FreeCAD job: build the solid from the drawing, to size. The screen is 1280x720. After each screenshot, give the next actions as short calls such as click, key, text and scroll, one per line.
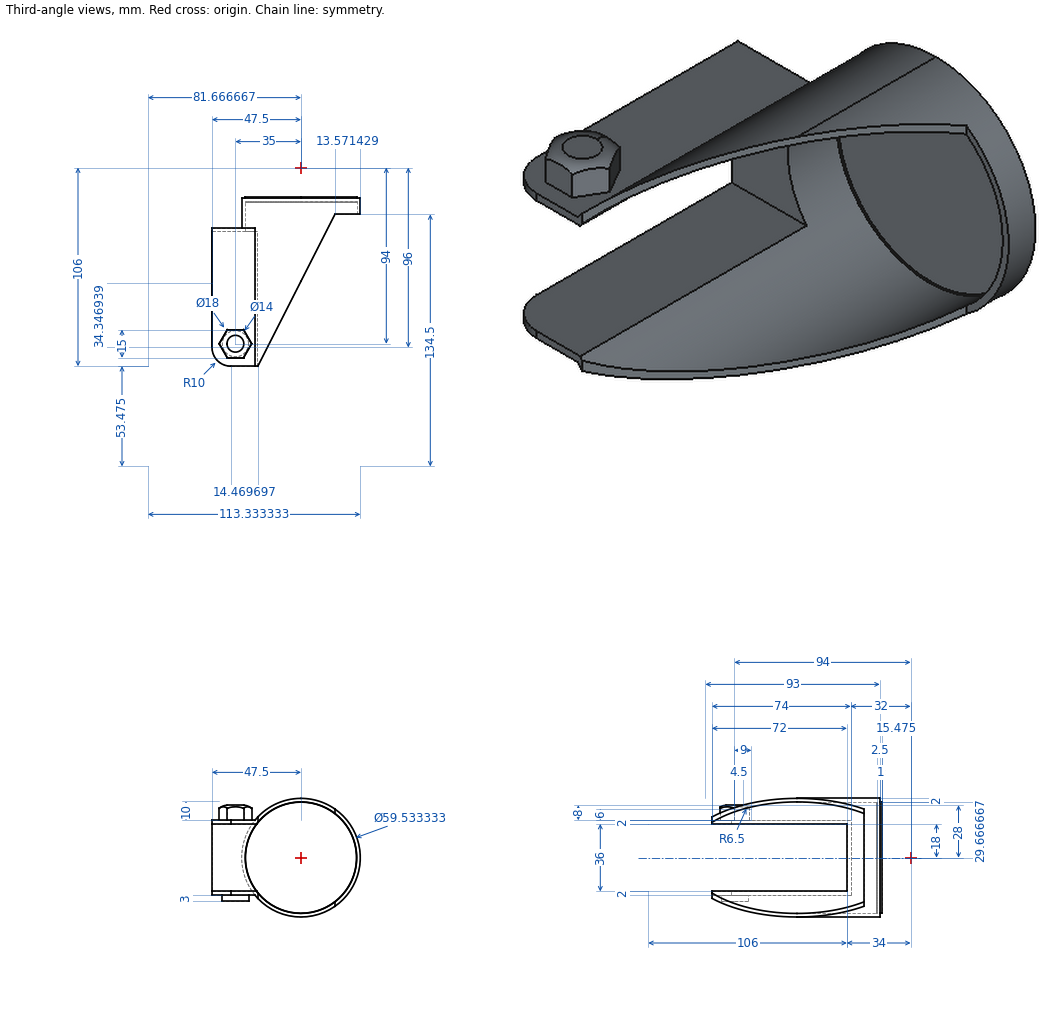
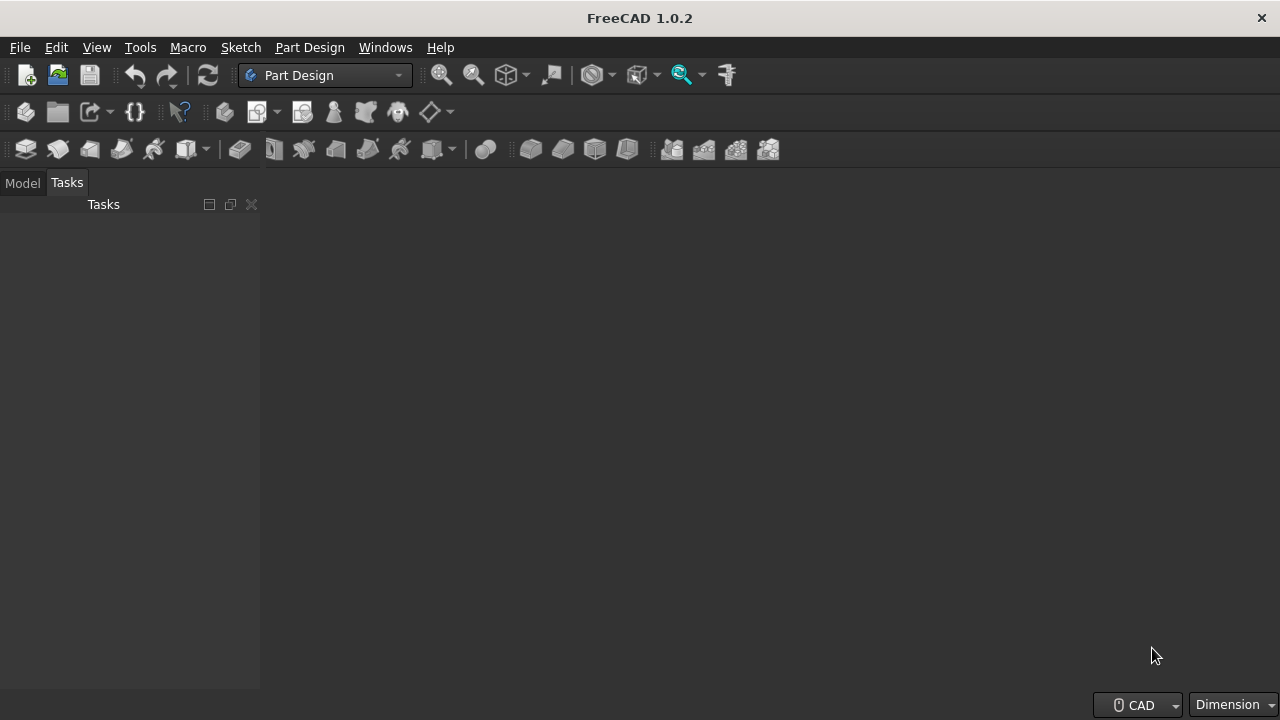
key(ctrl+n)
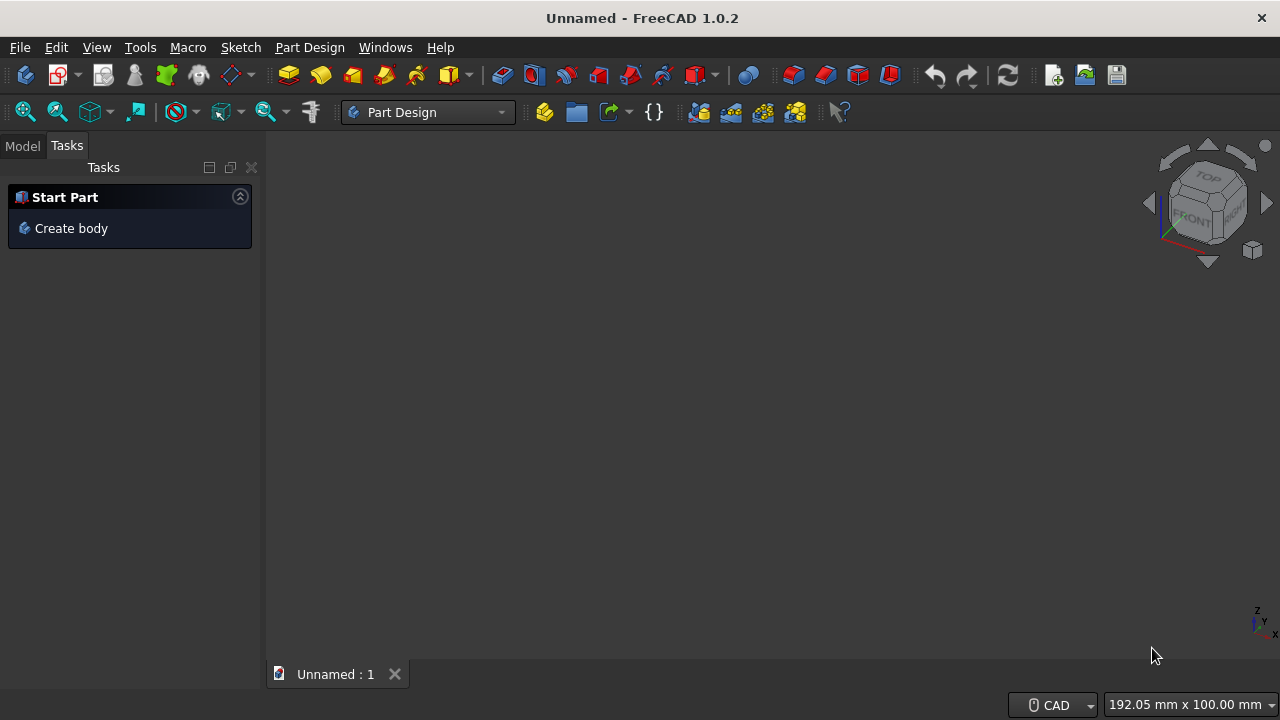
click(58, 76)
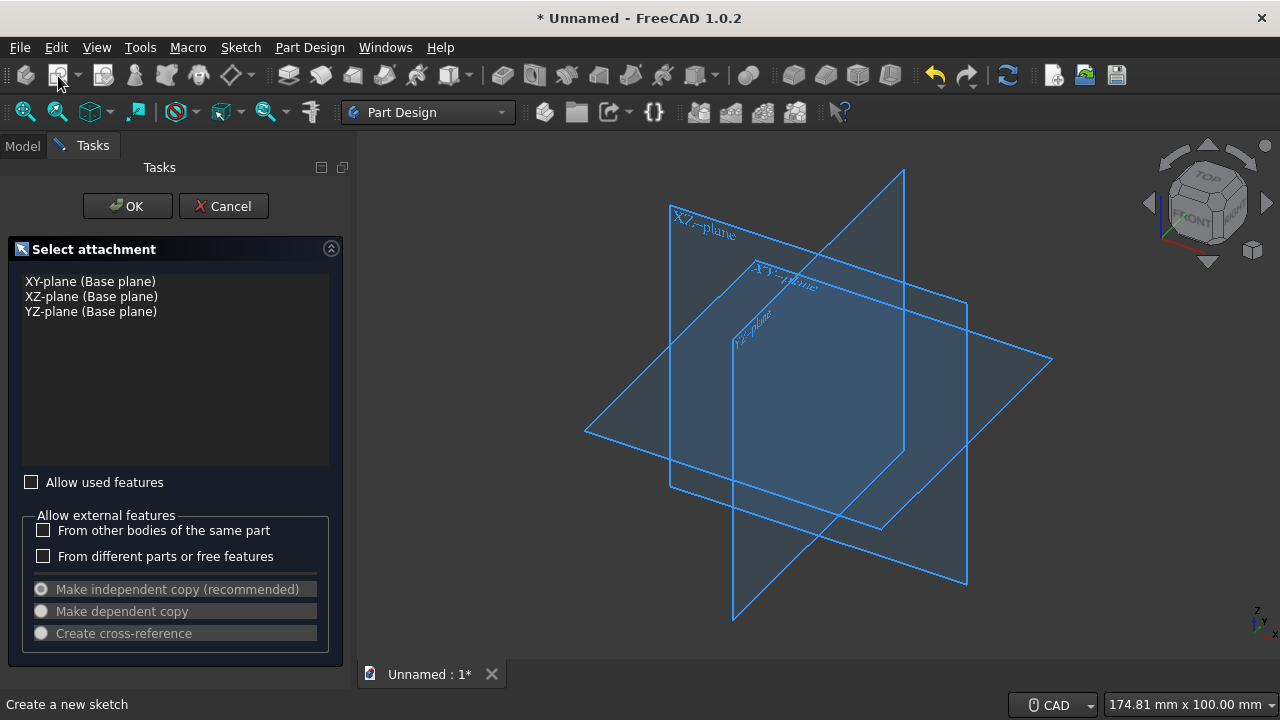
click(82, 312)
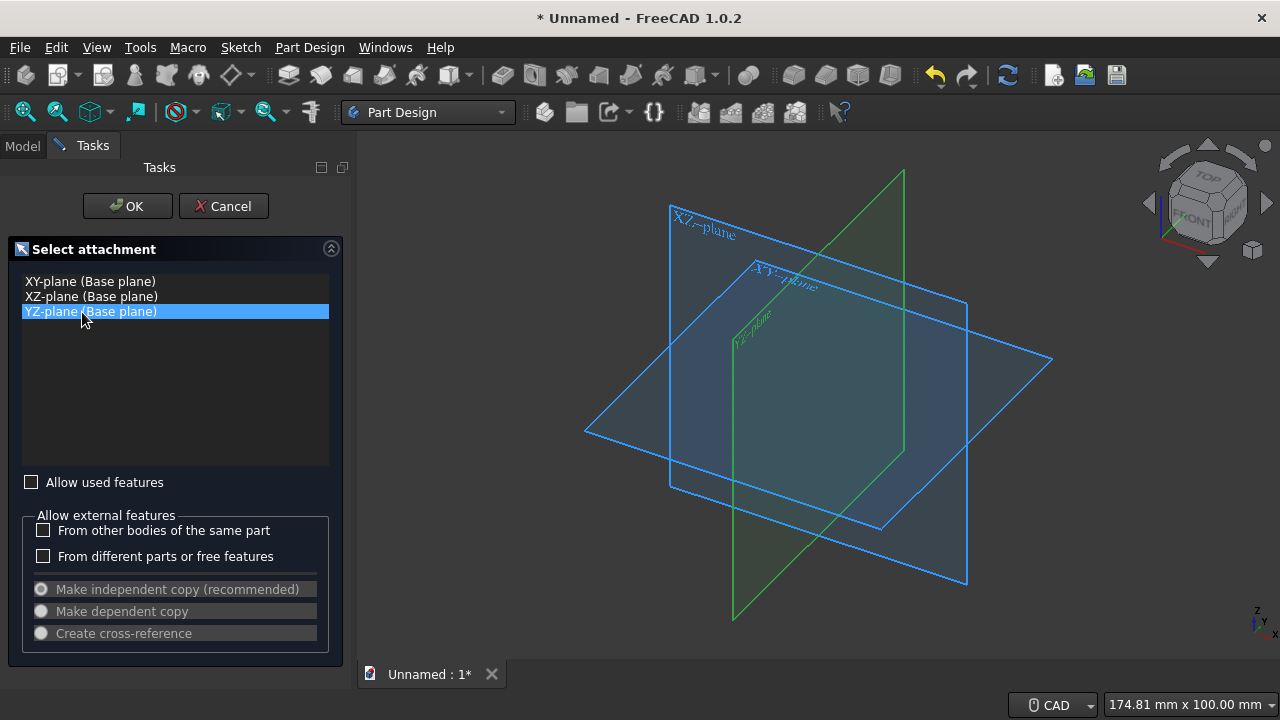
click(128, 206)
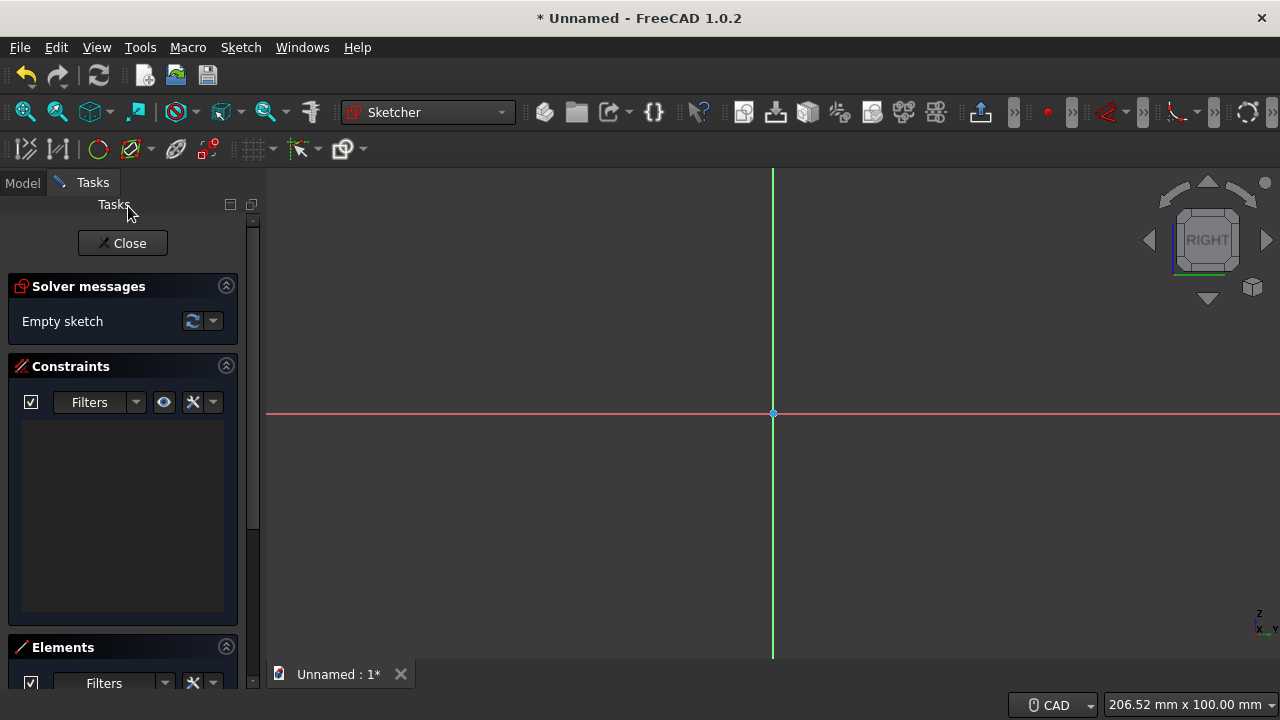
scroll(1115, 631, down, 1)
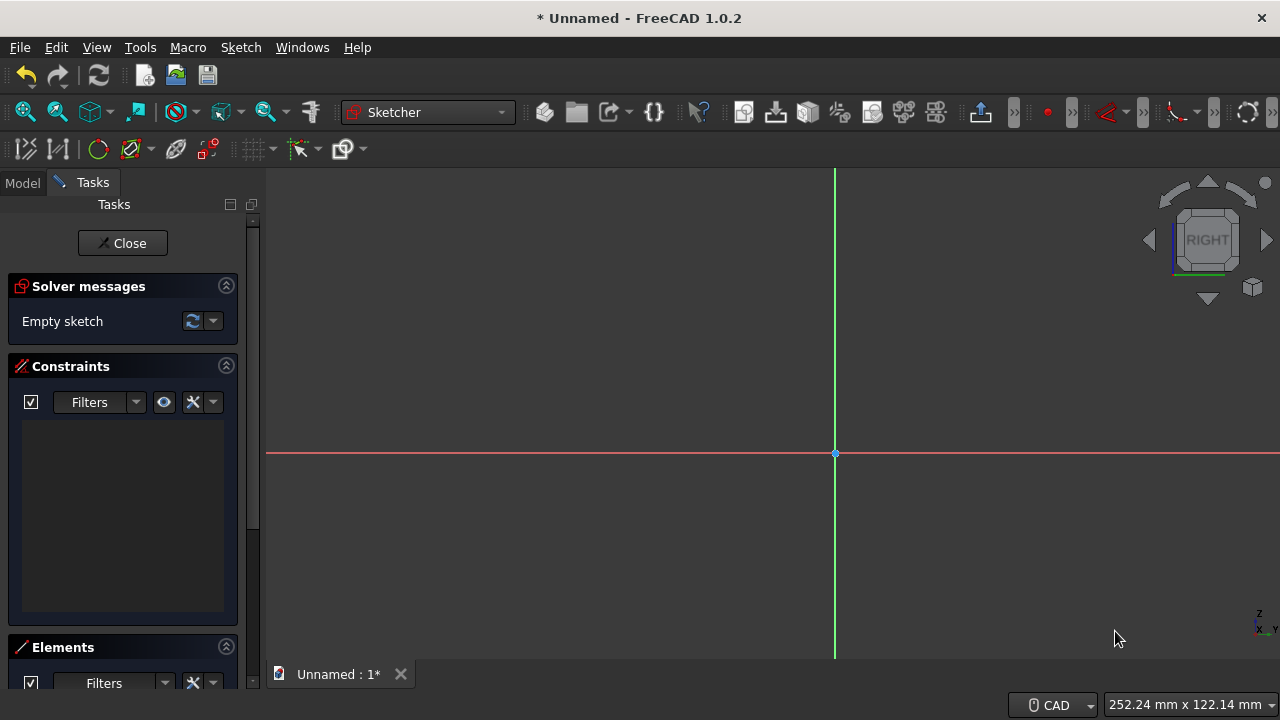
key(g)
key(m)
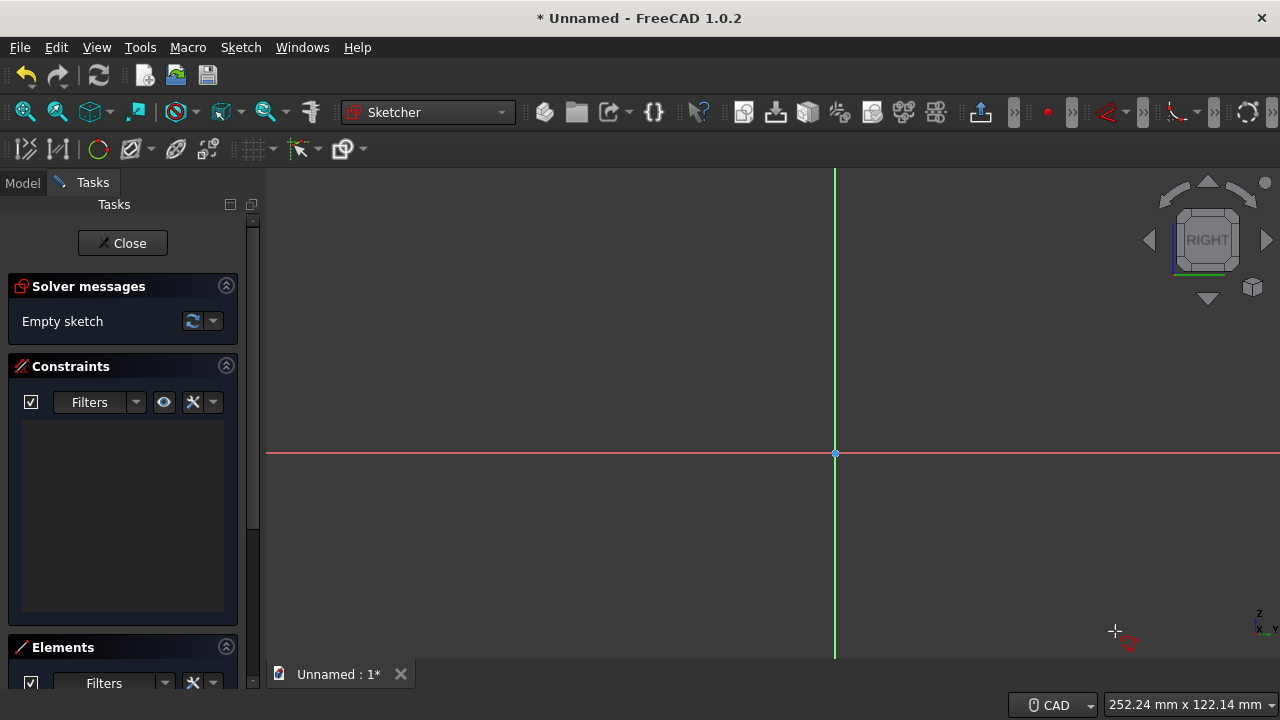
click(773, 453)
click(773, 334)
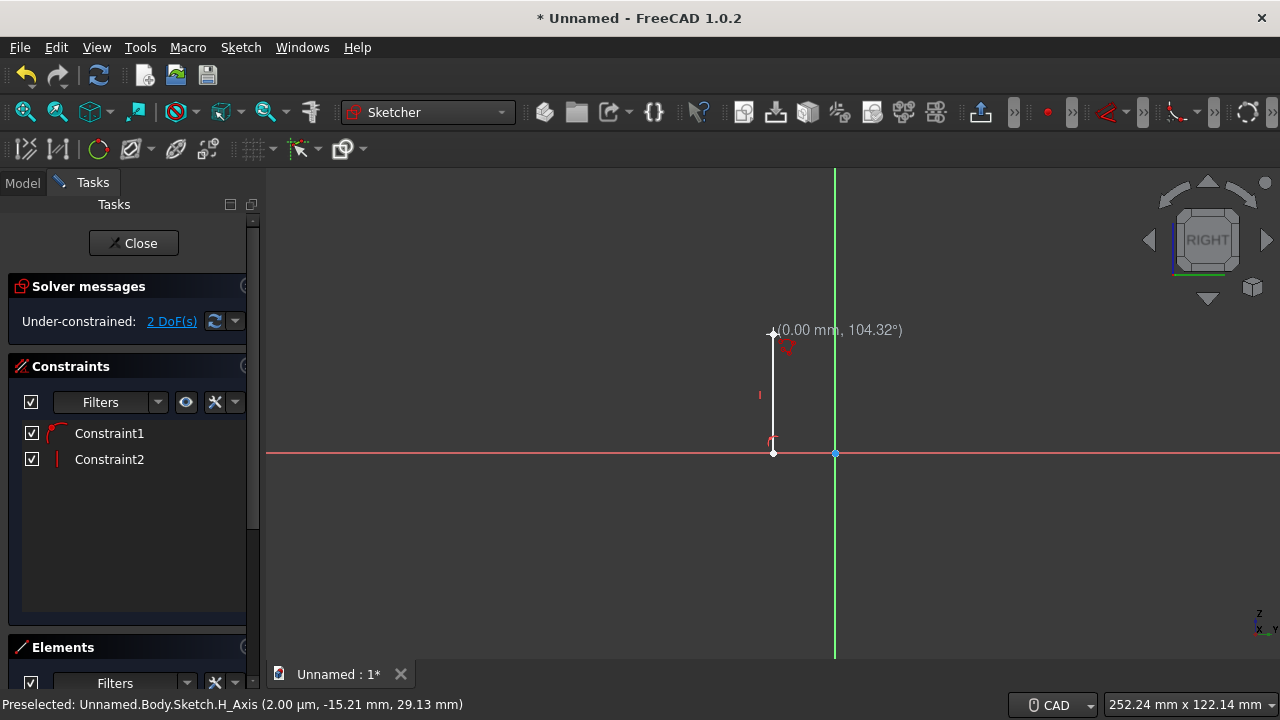
scroll(769, 334, up, 7)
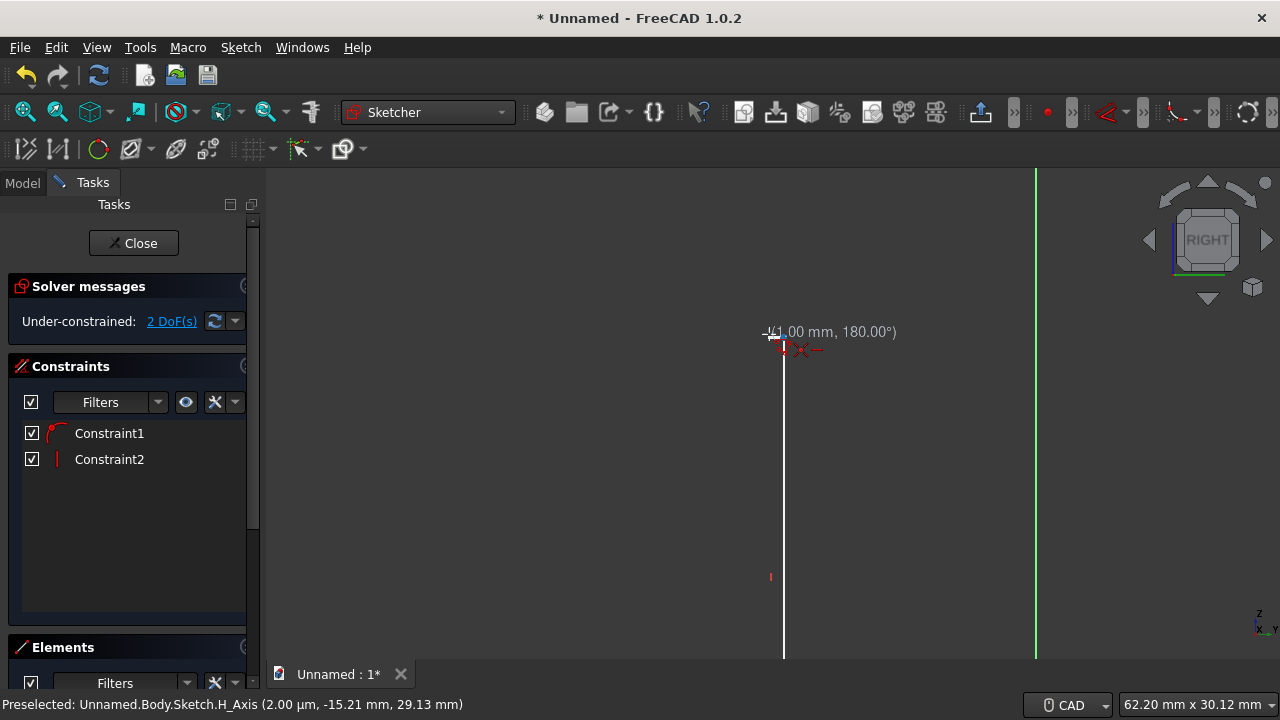
click(767, 333)
click(767, 300)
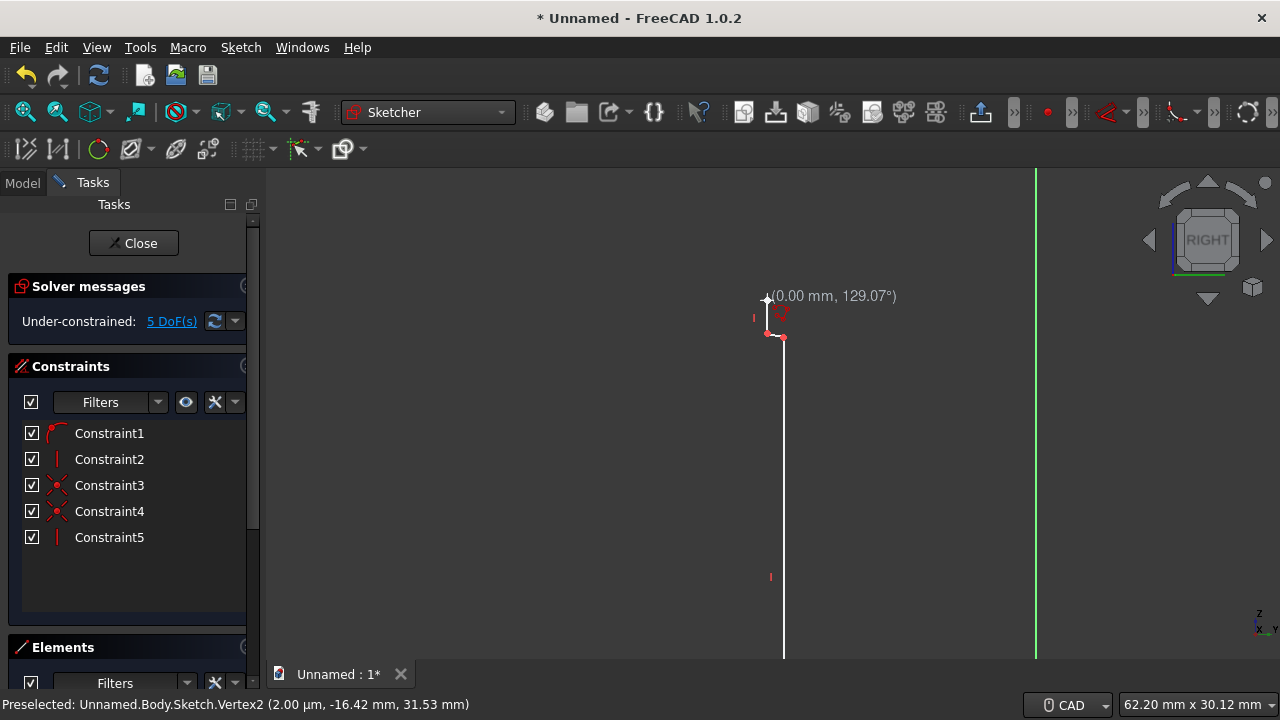
scroll(946, 351, down, 6)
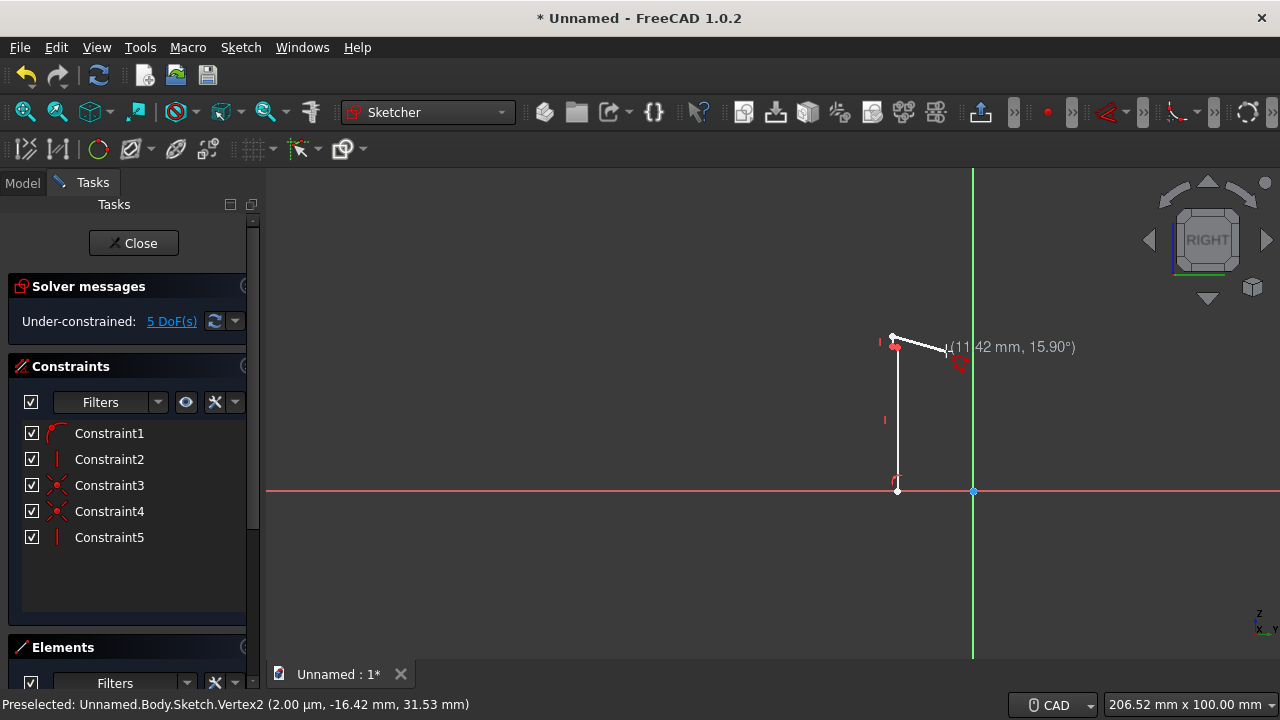
click(436, 336)